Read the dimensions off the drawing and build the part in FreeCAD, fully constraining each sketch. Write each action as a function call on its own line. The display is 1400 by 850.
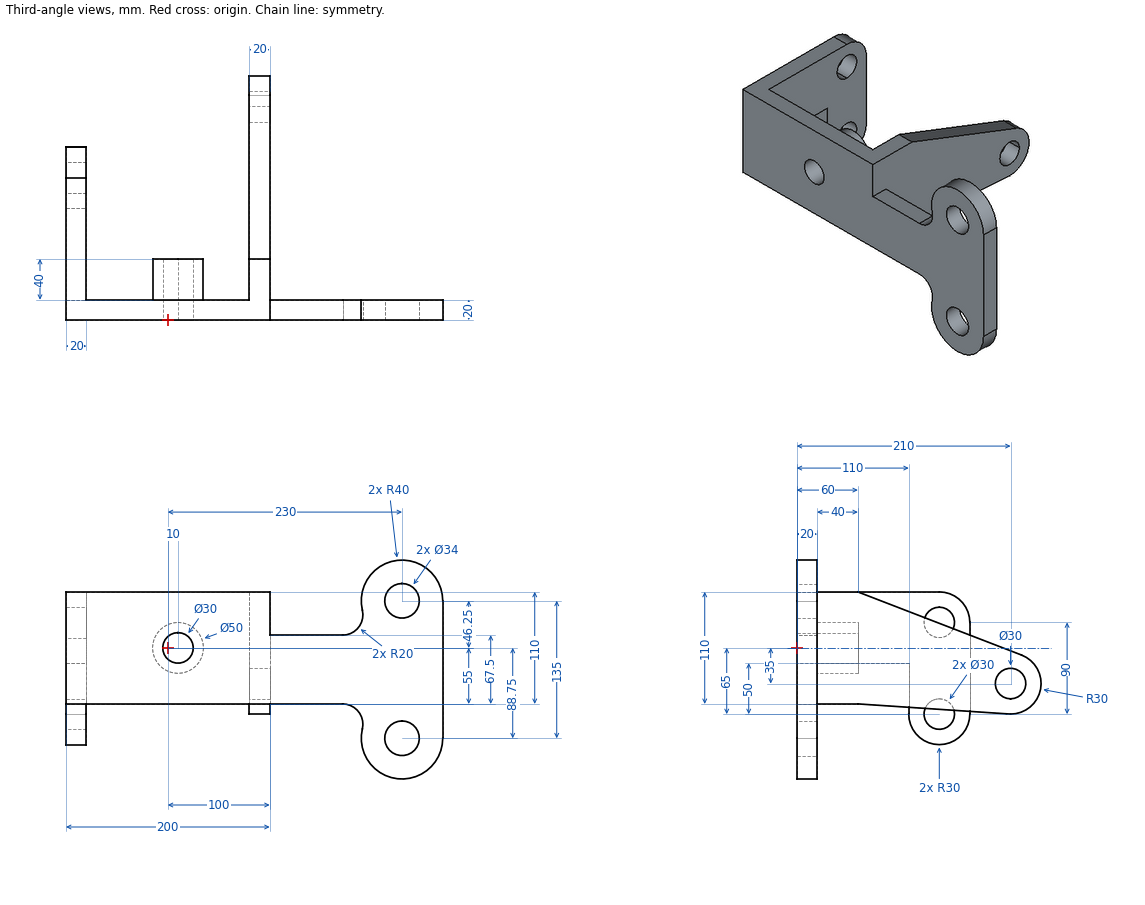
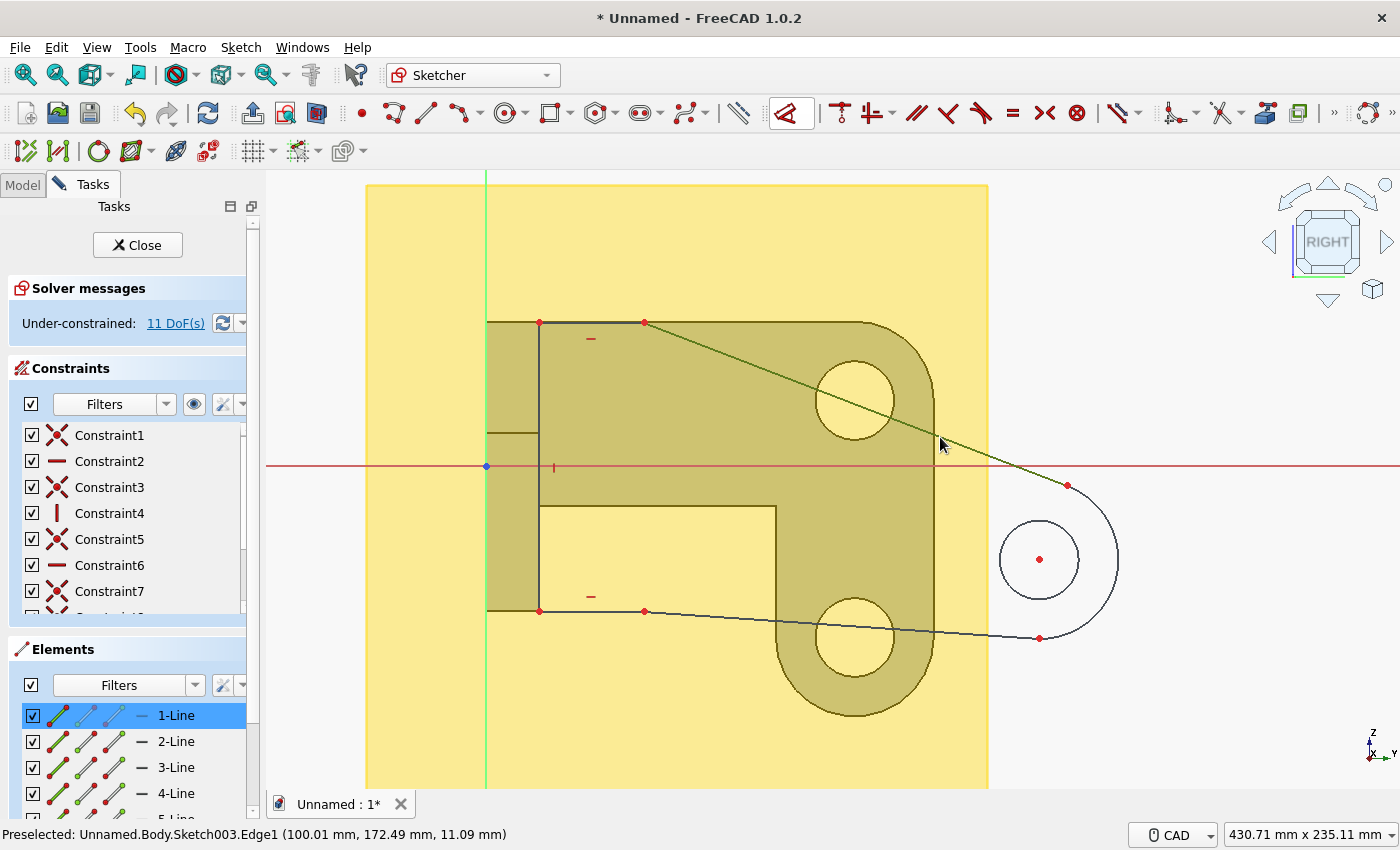
click(1098, 613)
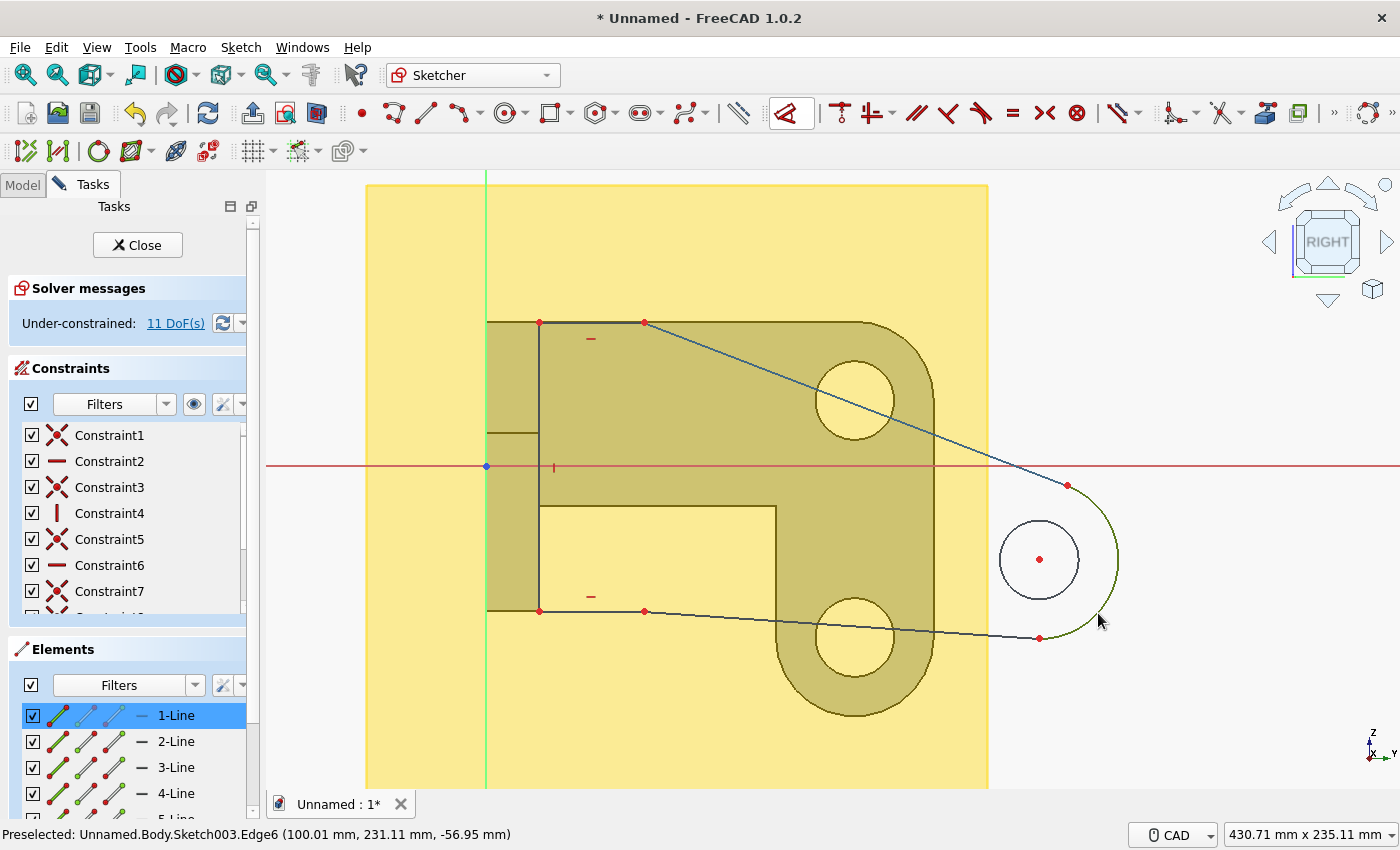
click(982, 114)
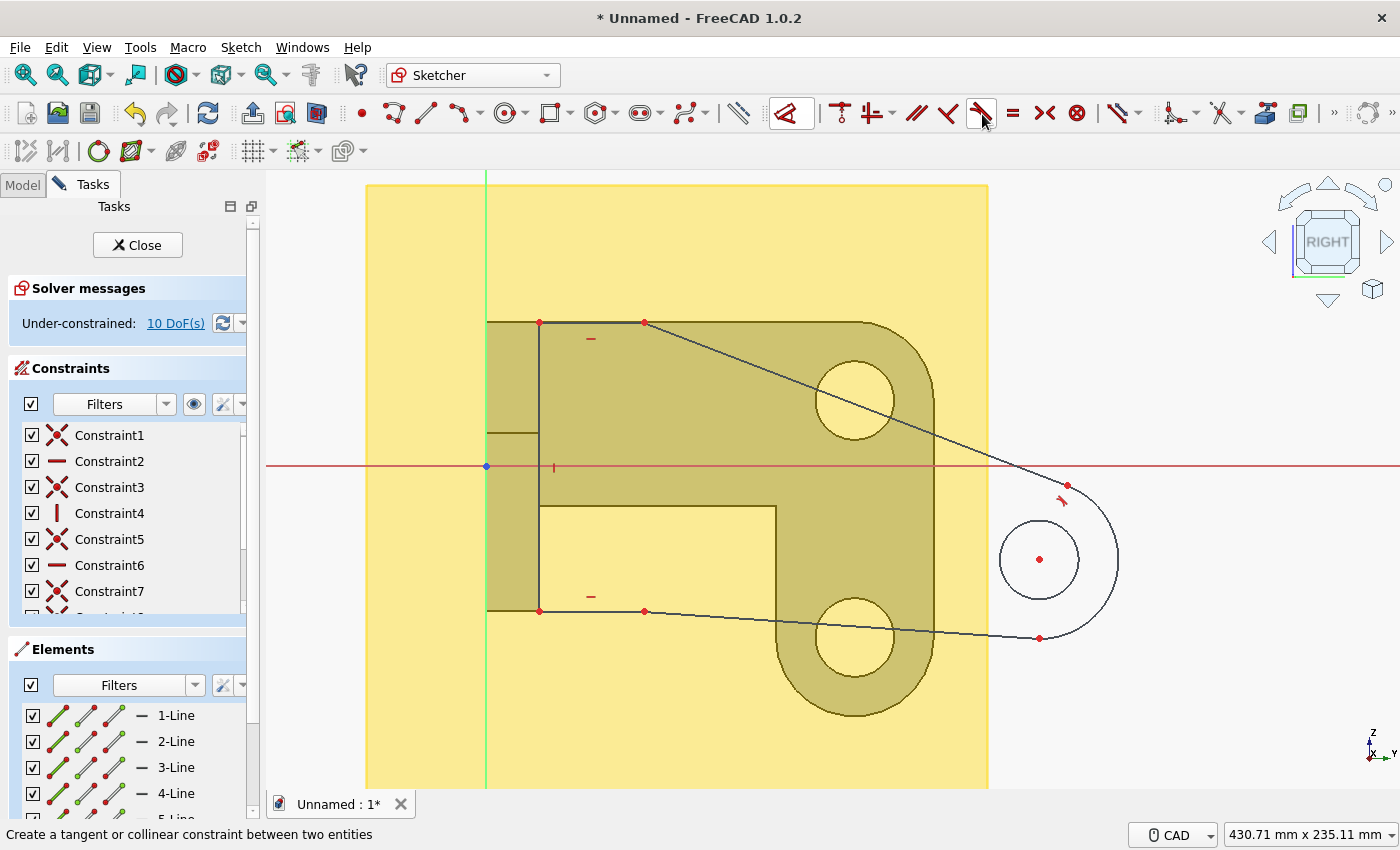
click(644, 323)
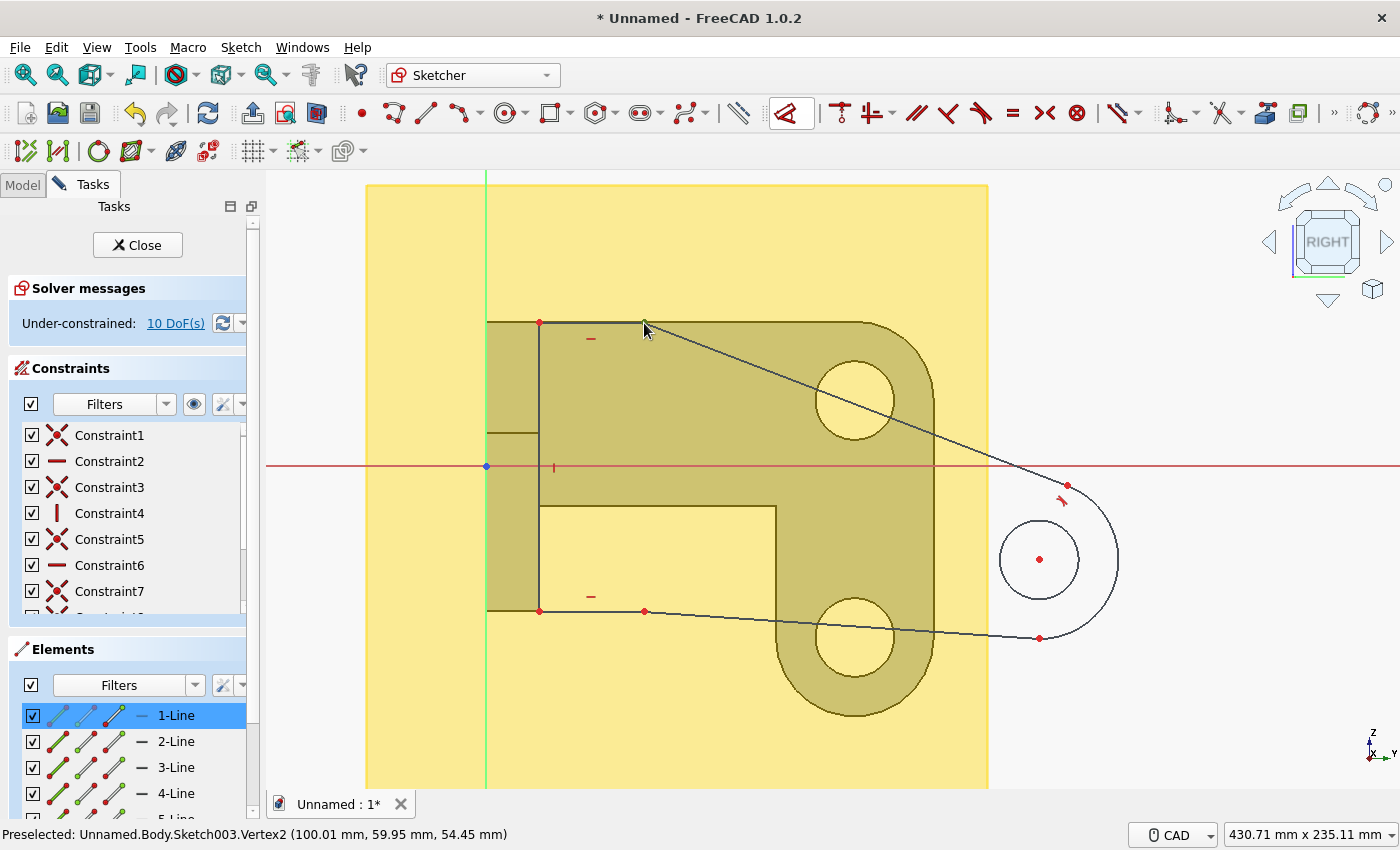
click(644, 612)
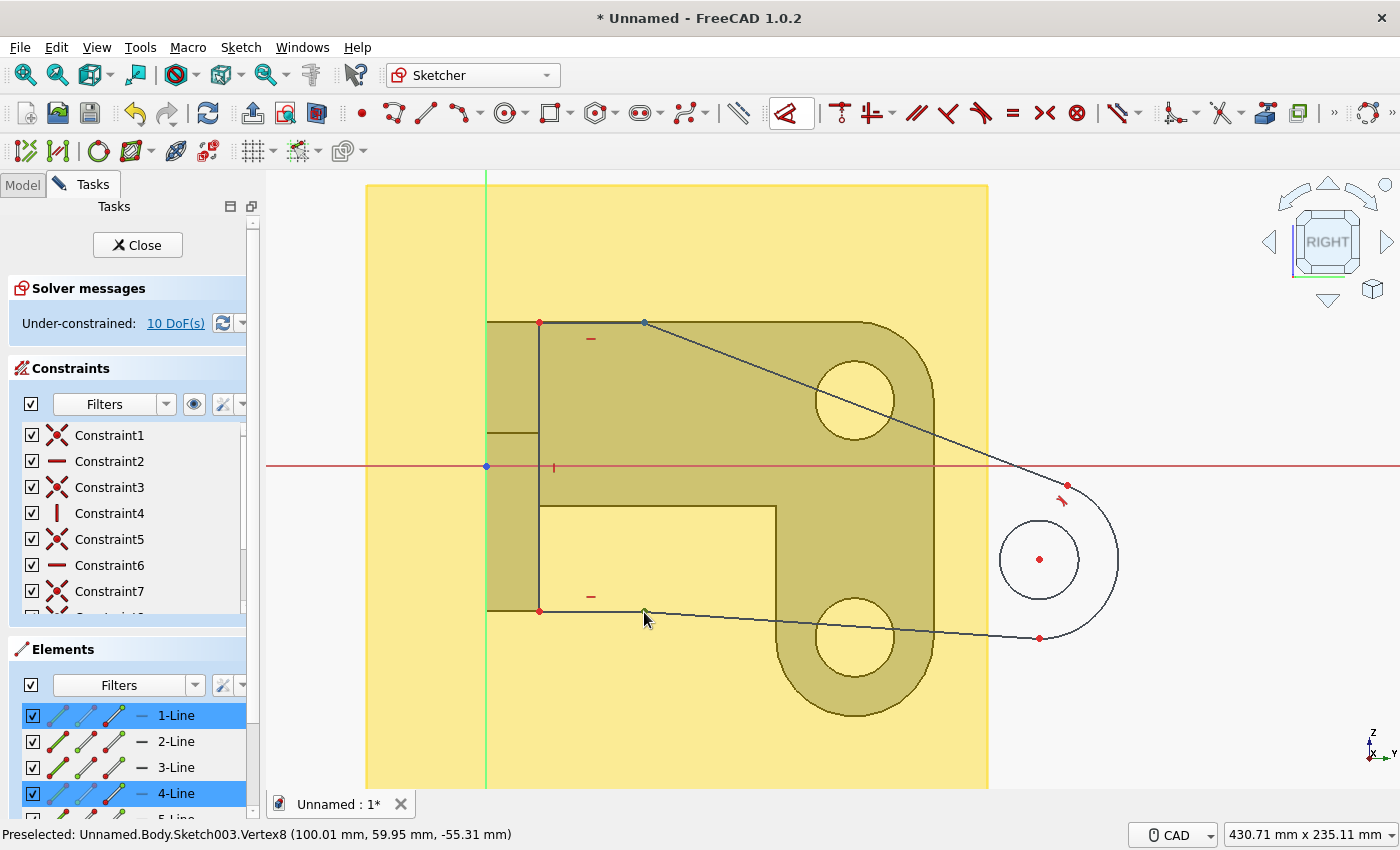
click(361, 466)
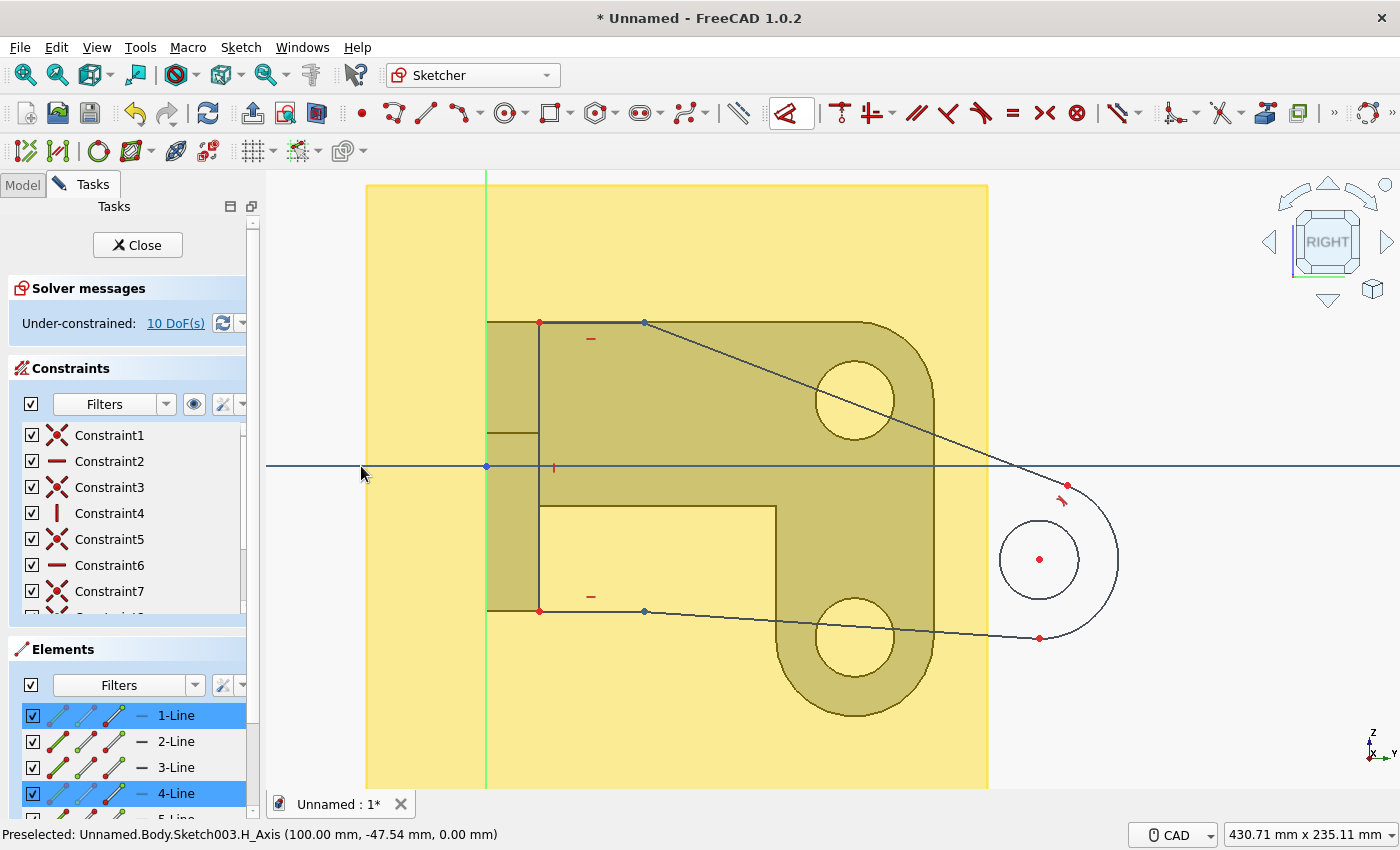
key(s)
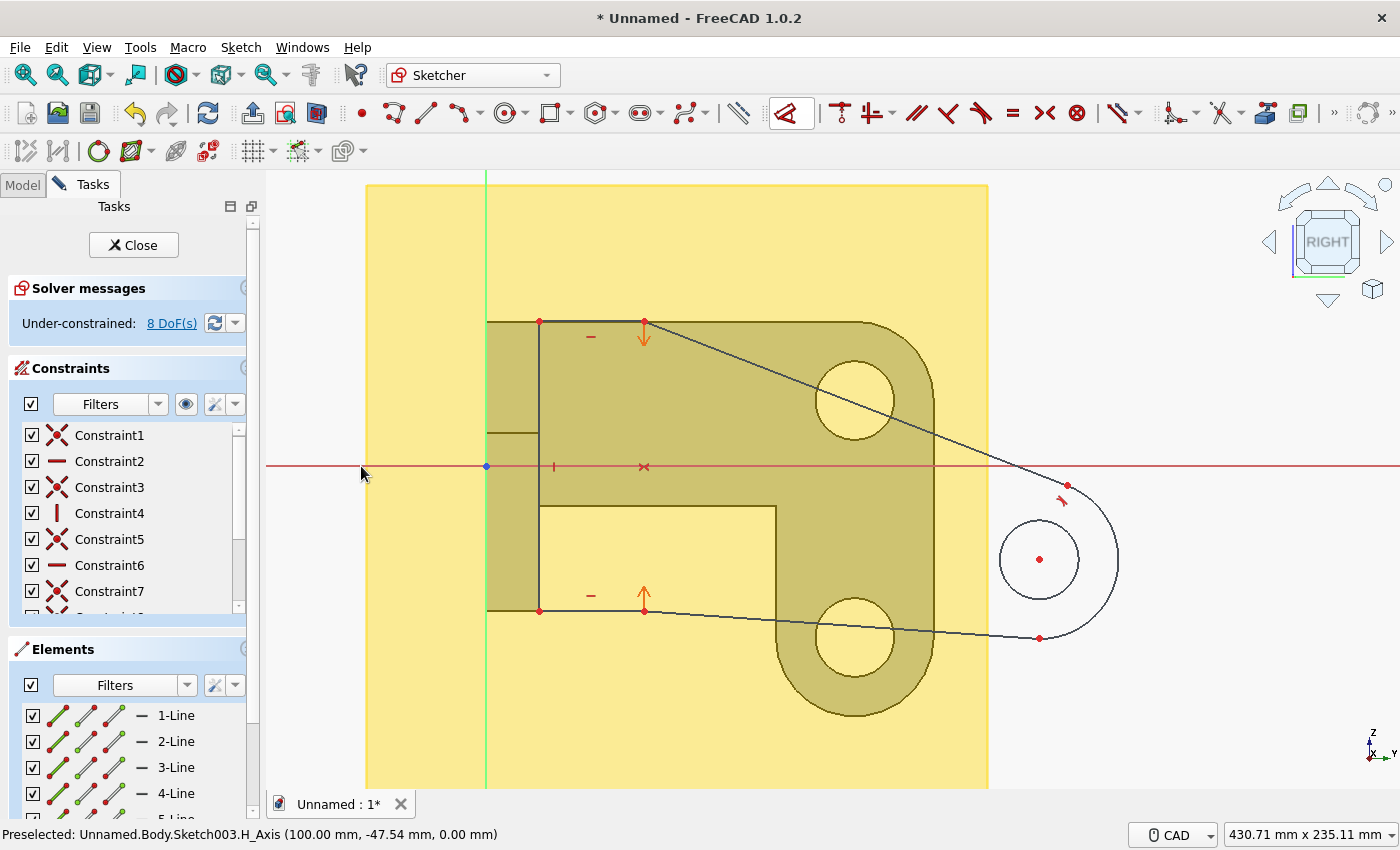
click(1098, 613)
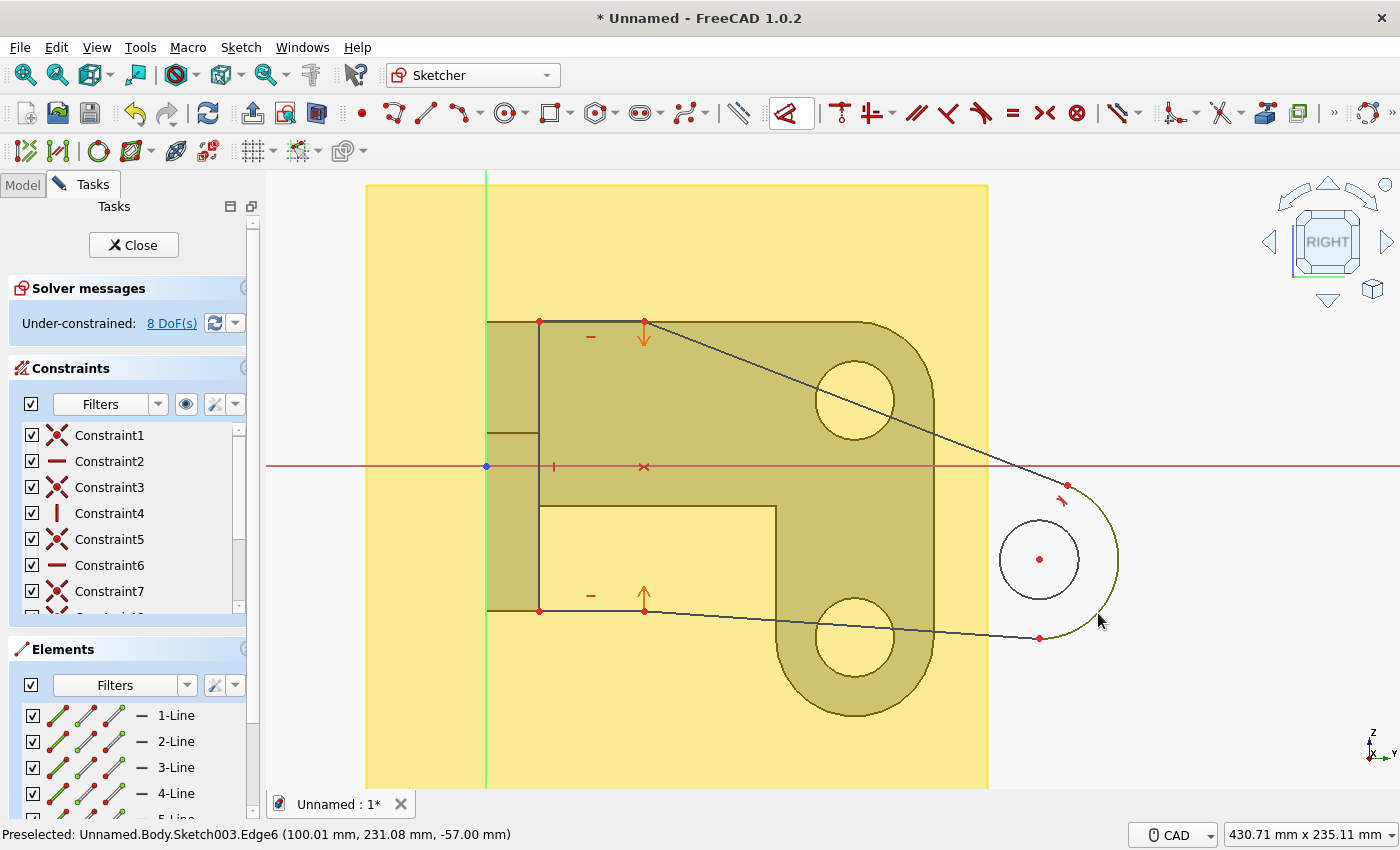
key(k)
key(r)